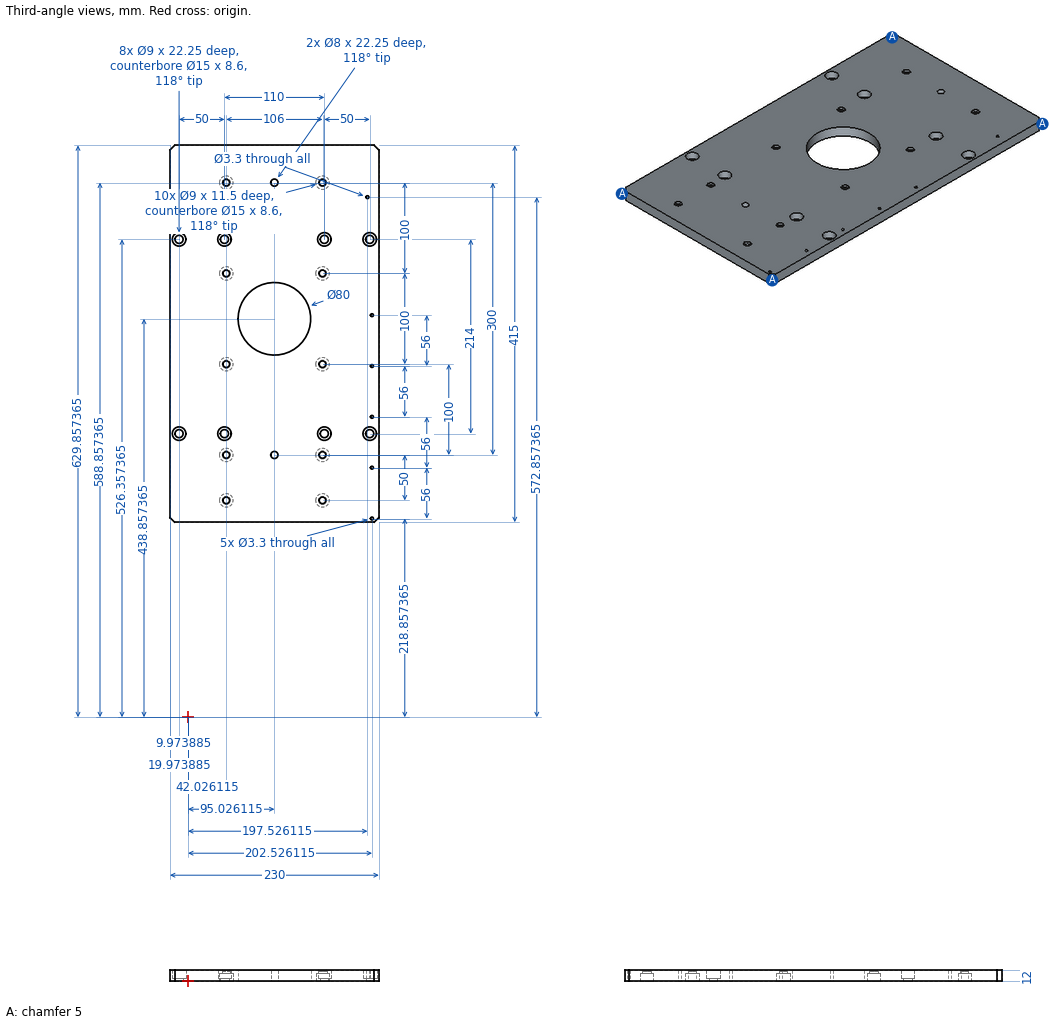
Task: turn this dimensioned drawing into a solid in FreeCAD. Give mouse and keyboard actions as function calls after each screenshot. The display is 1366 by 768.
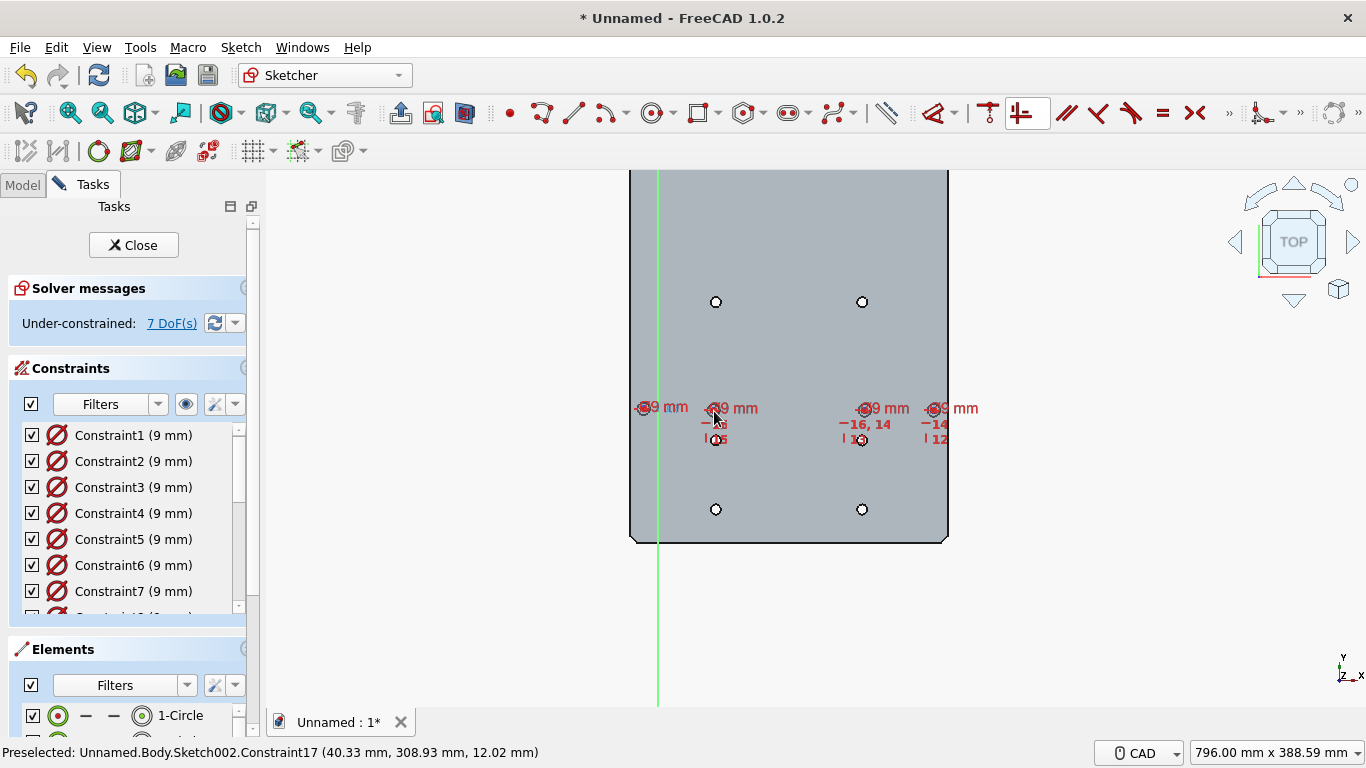
click(714, 410)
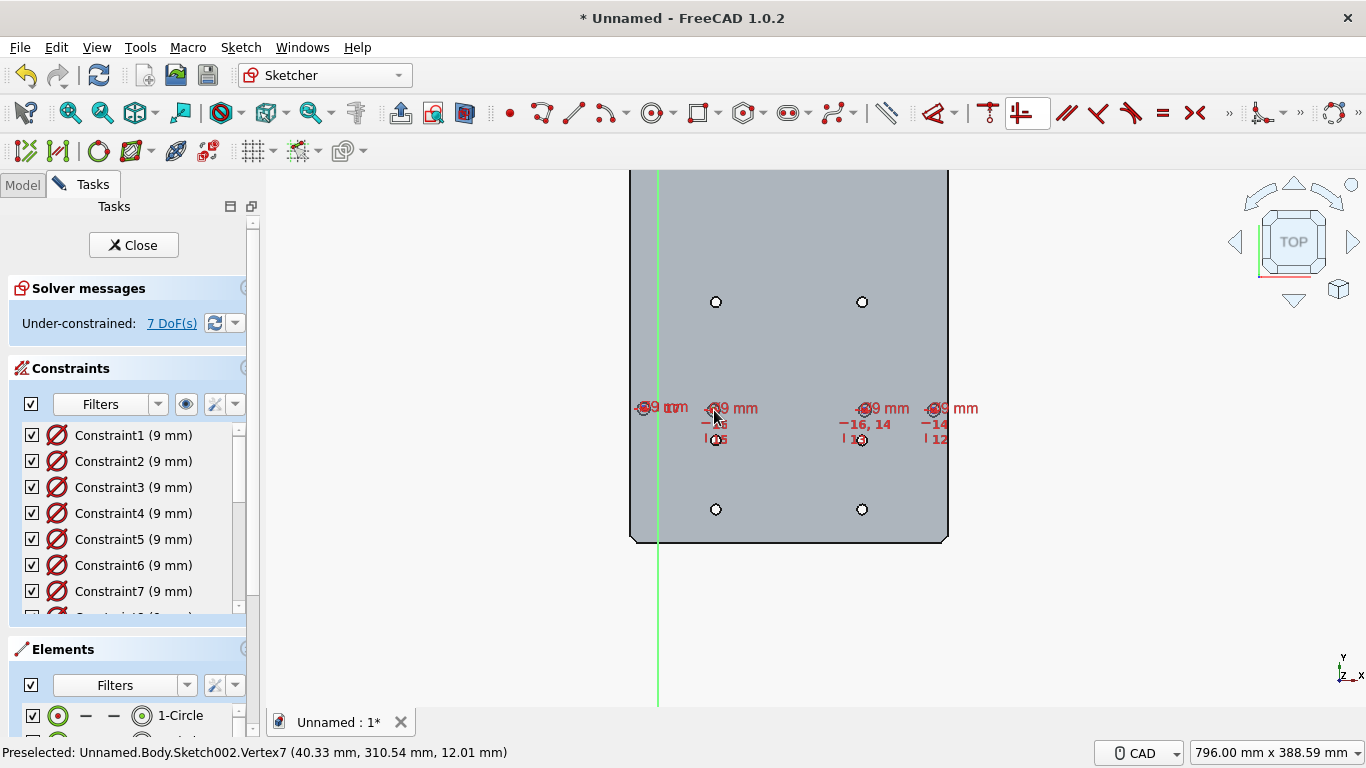
click(644, 409)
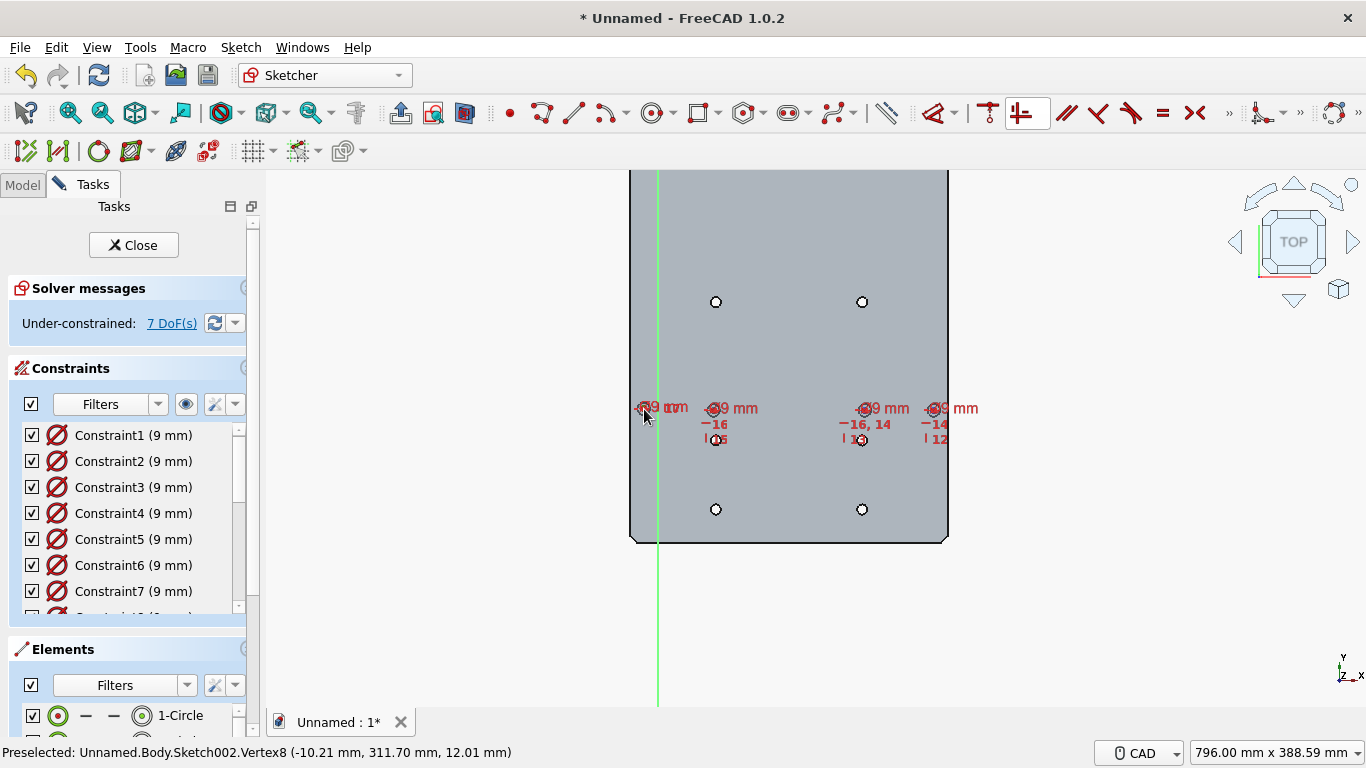
key(h)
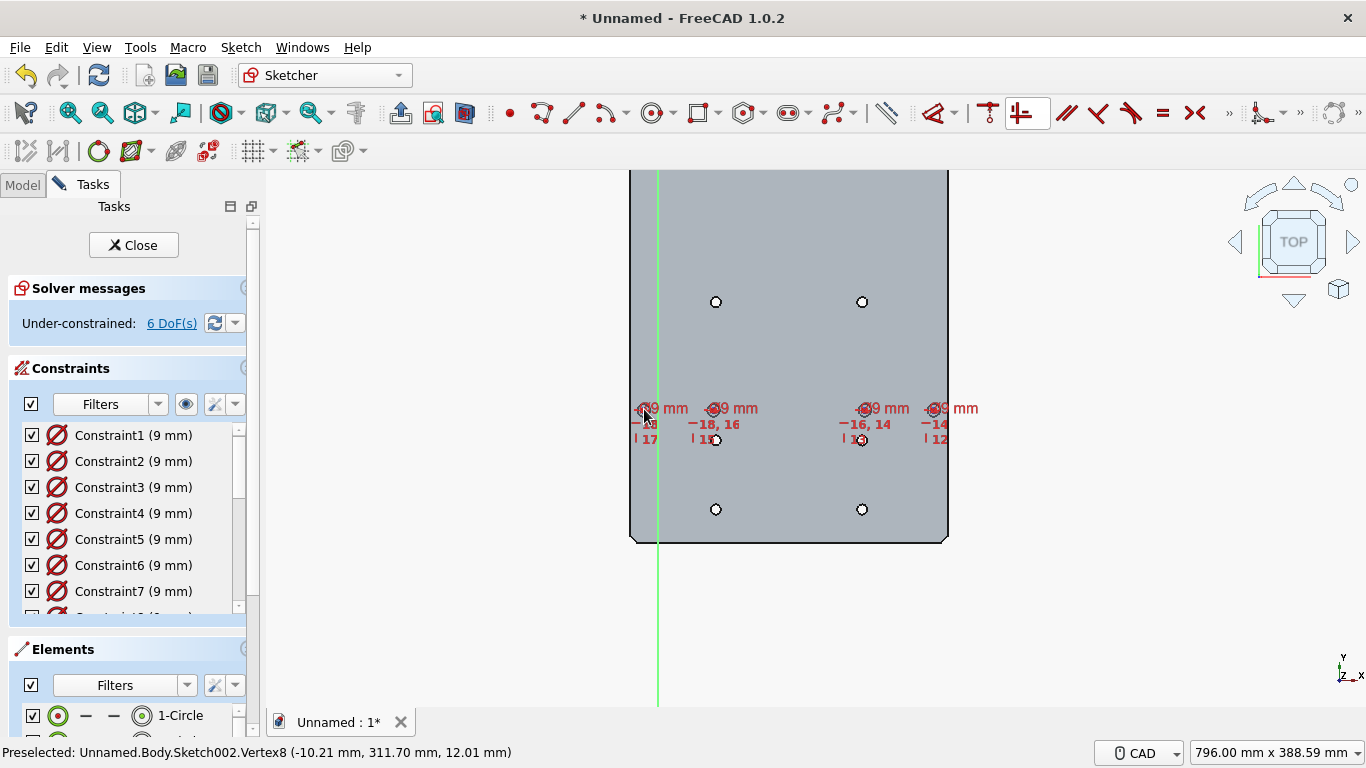
click(934, 114)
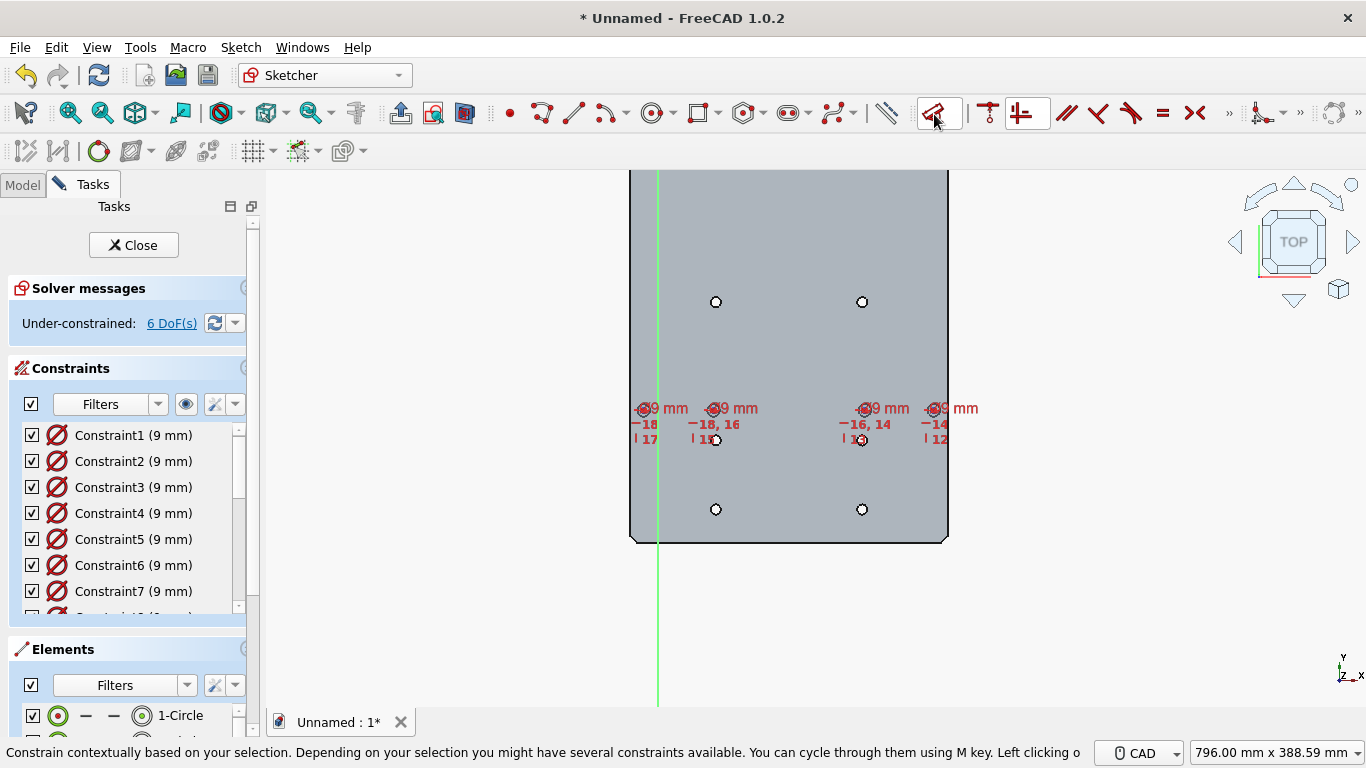
scroll(714, 411, down, 4)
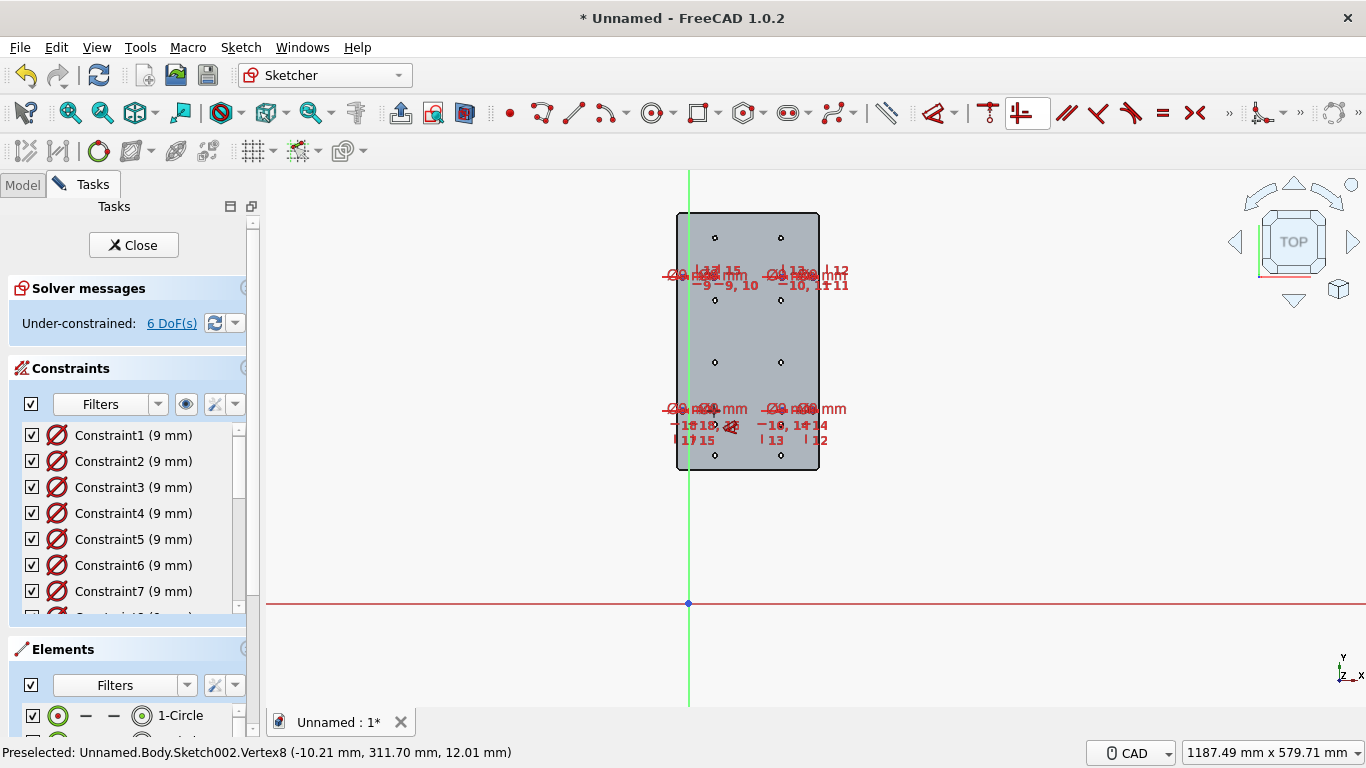
scroll(683, 277, up, 2)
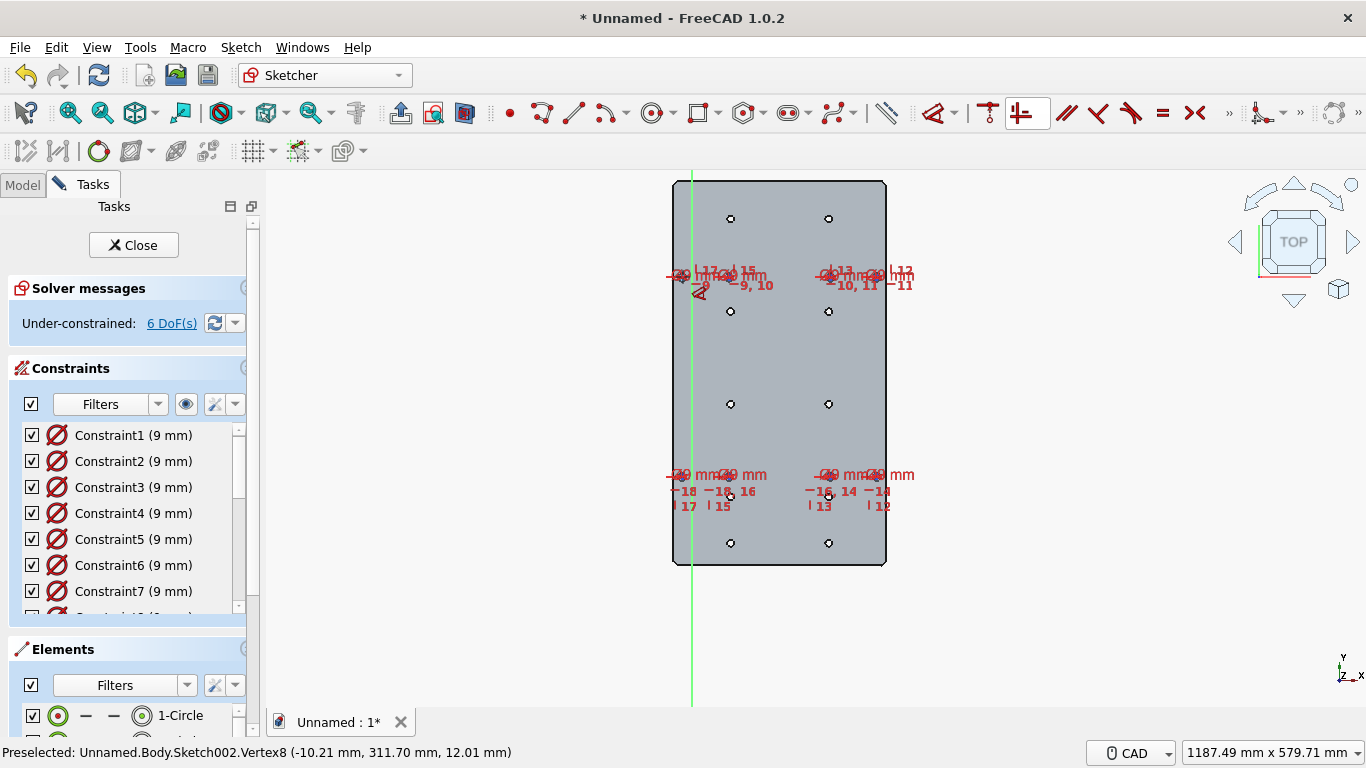
click(682, 277)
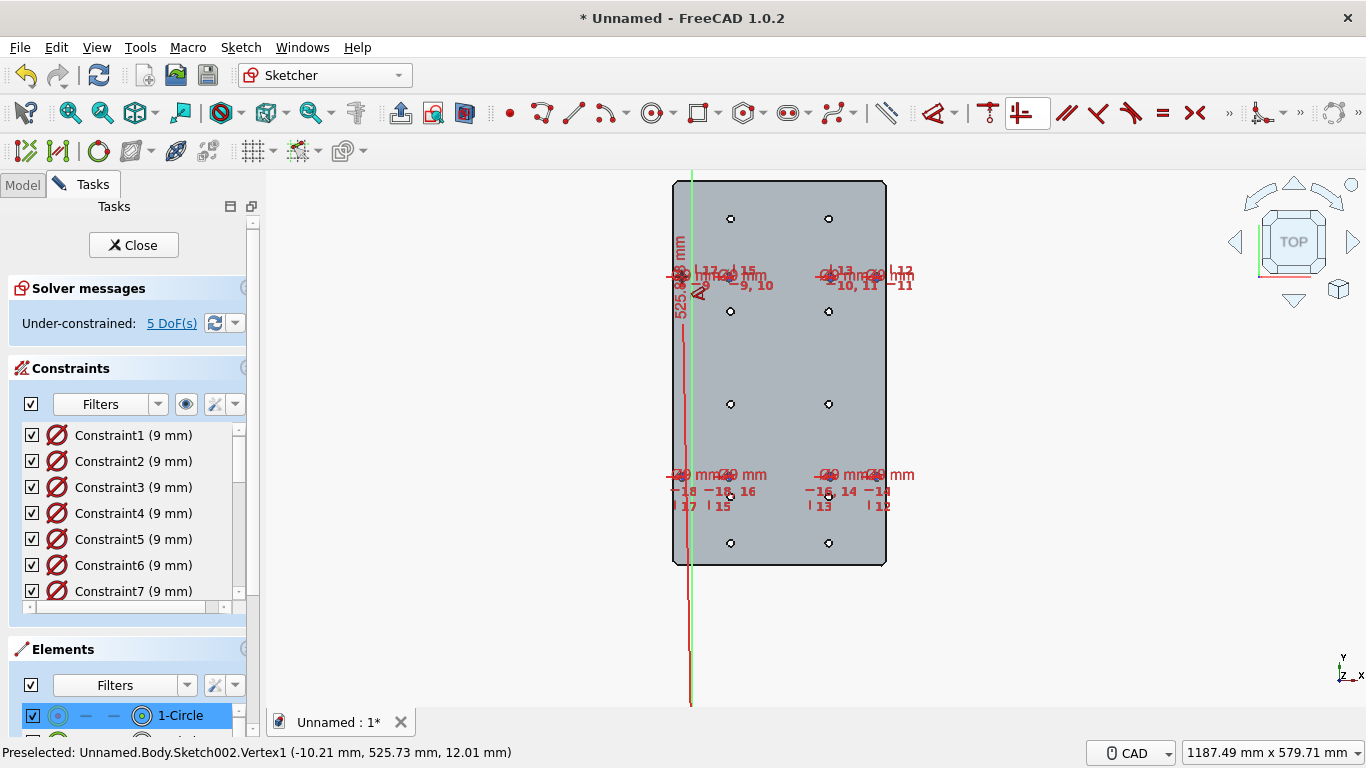
click(729, 277)
click(706, 243)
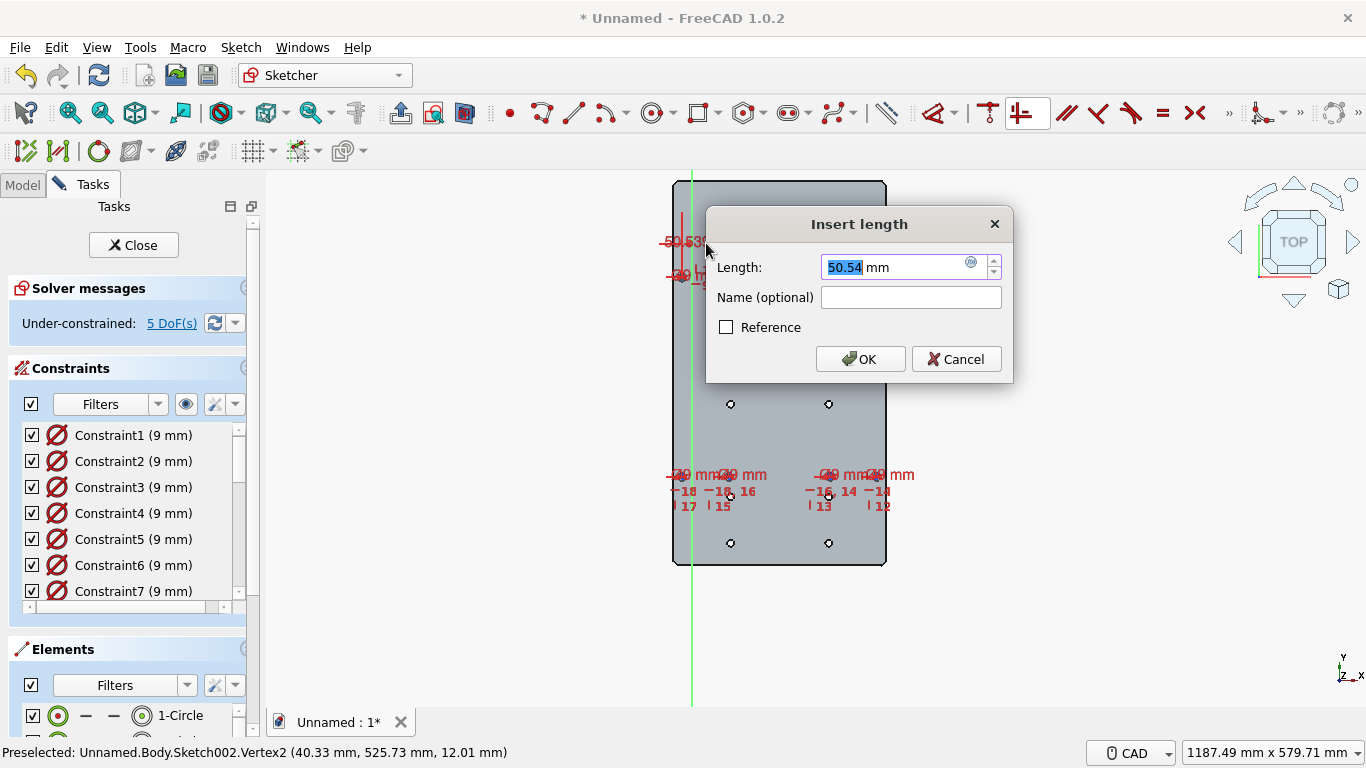
text(50)
key(Return)